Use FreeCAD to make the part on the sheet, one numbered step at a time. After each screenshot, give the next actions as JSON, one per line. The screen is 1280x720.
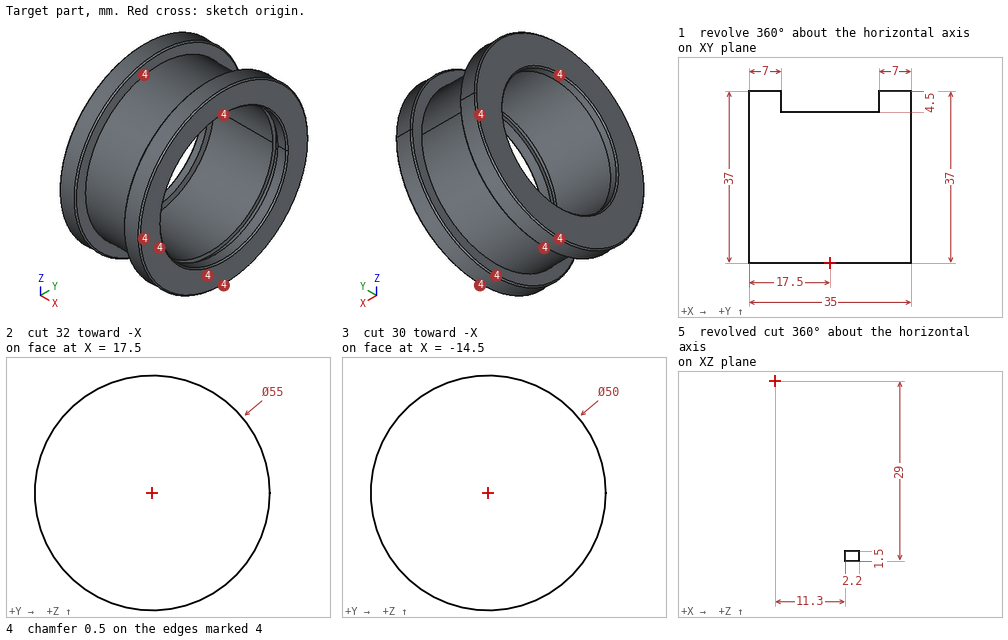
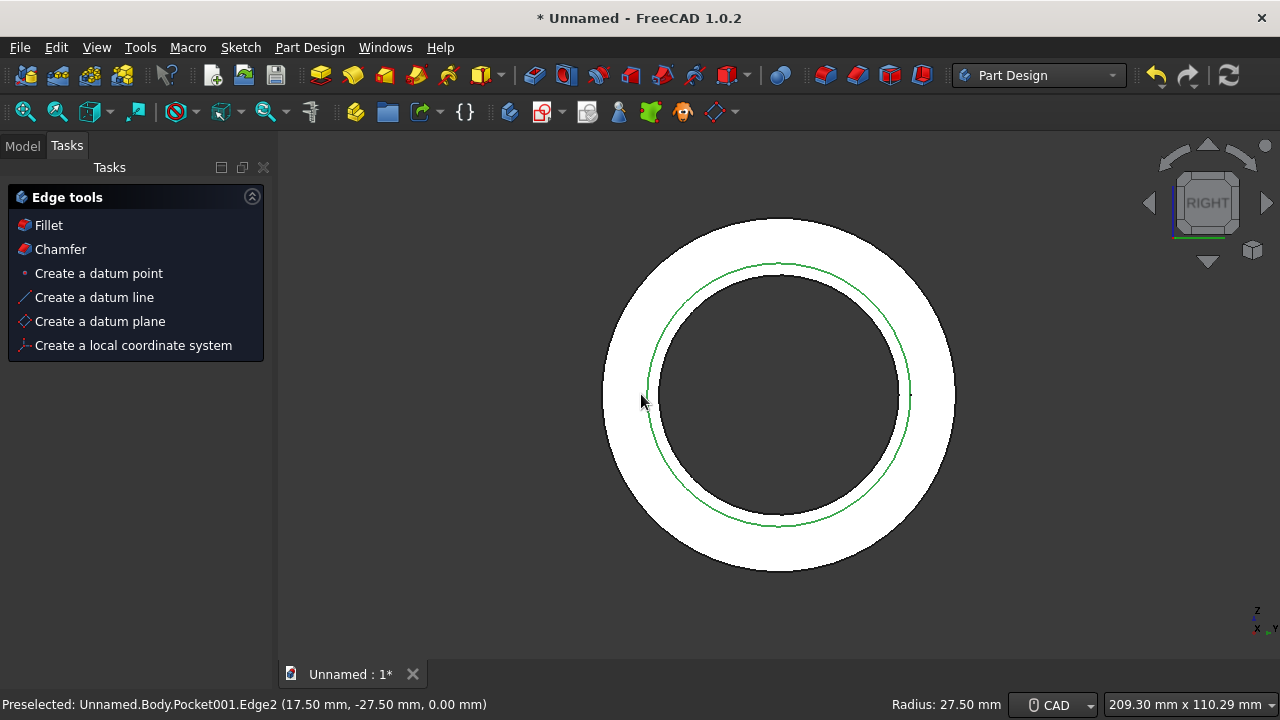
{"action": "left_click", "coordinate": [724, 562], "text": "ctrl"}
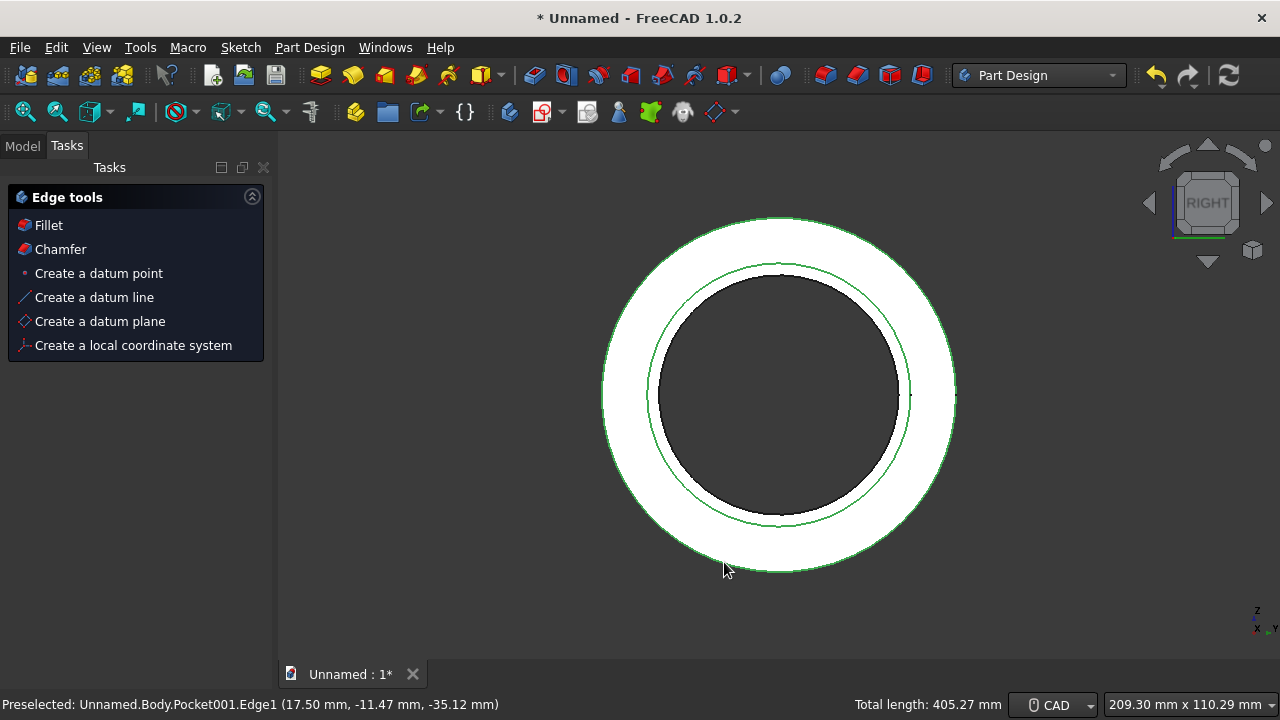
{"action": "key", "text": "0"}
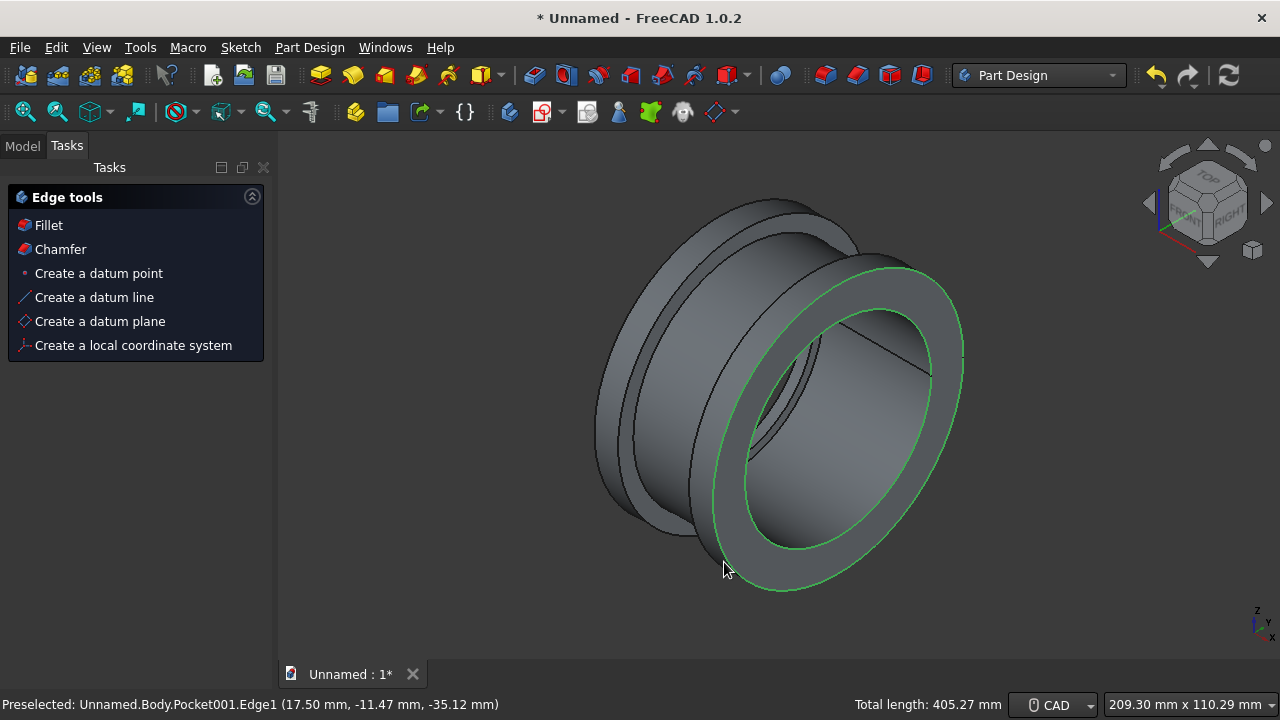
{"action": "left_click", "coordinate": [618, 446], "text": "ctrl"}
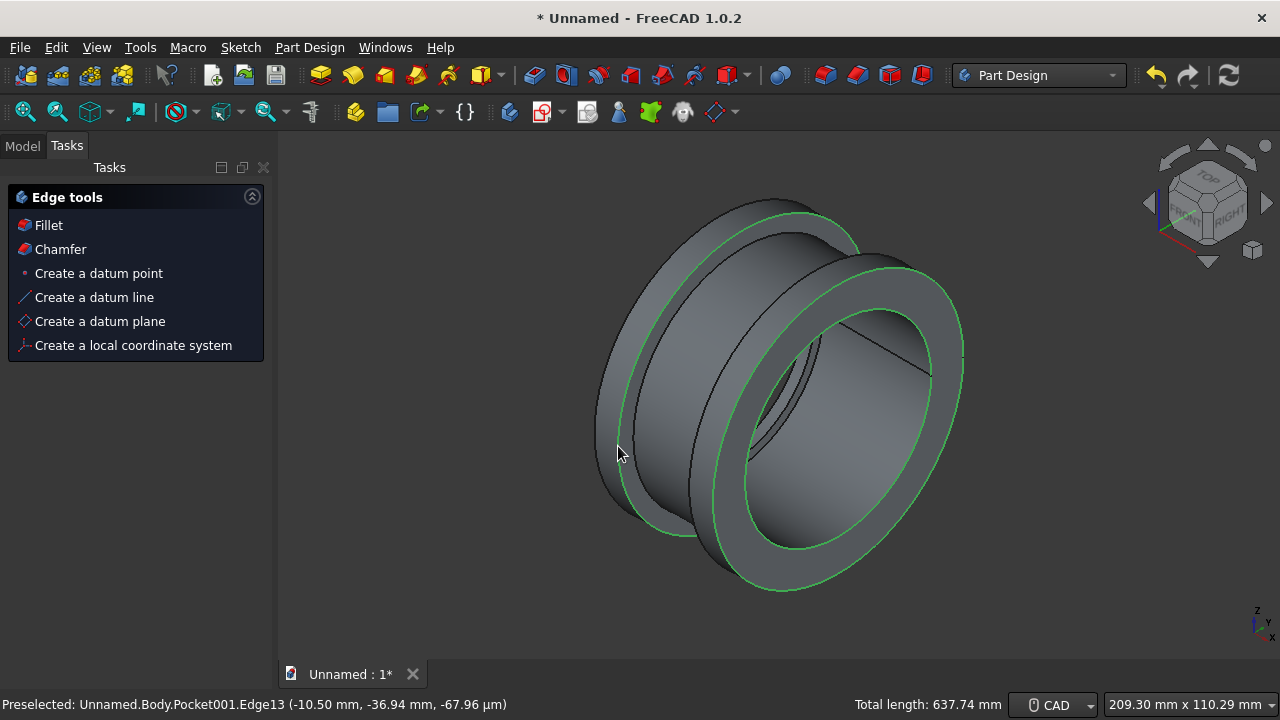
{"action": "key", "text": "2"}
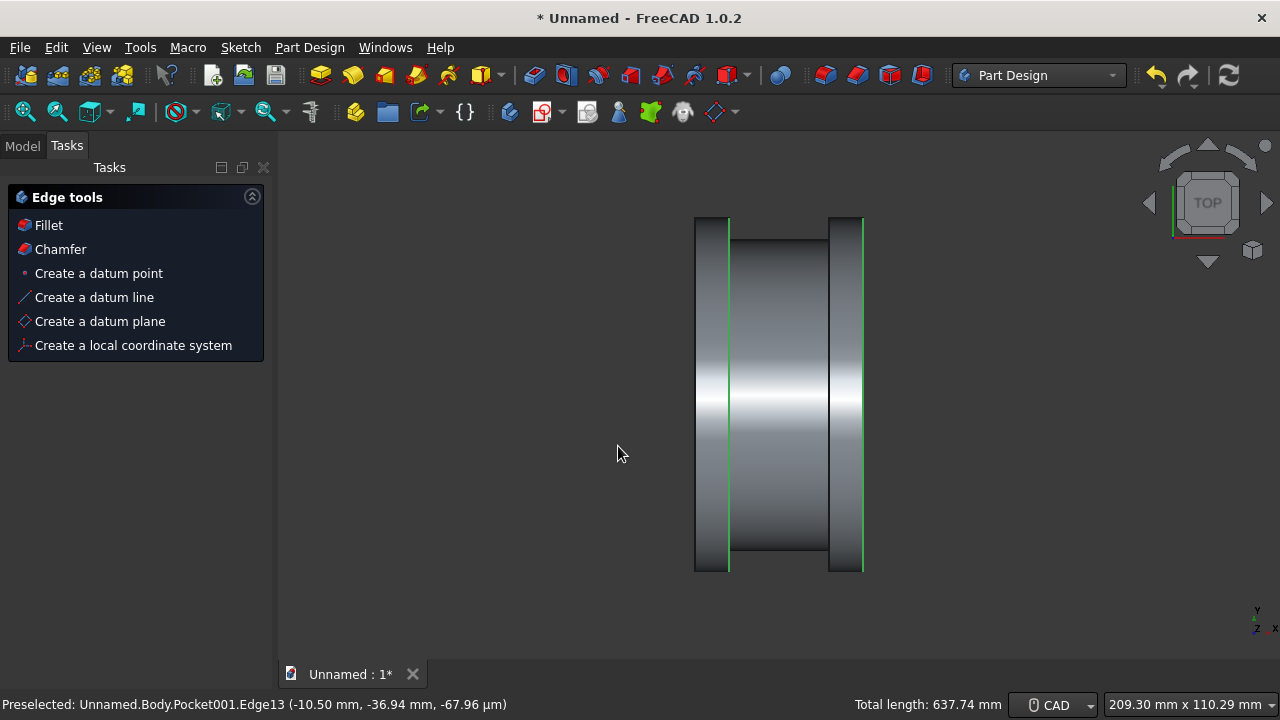
{"action": "left_click", "coordinate": [695, 537], "text": "ctrl"}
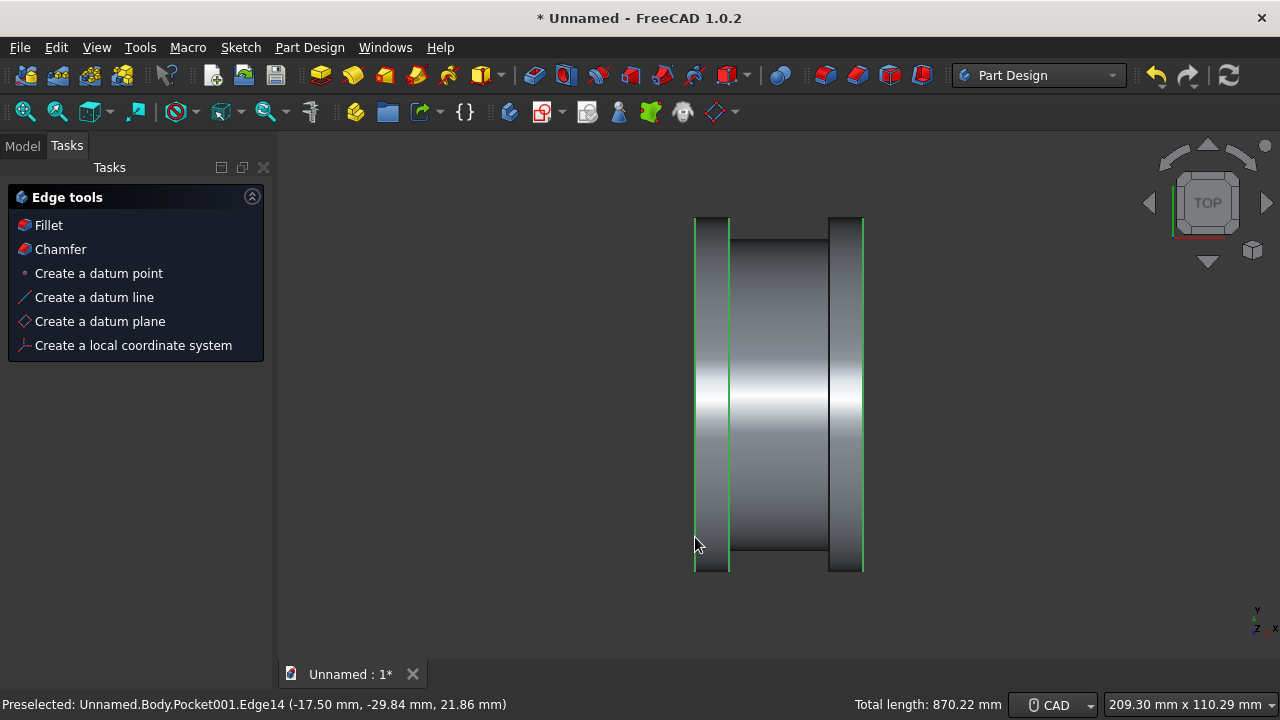
{"action": "left_click", "coordinate": [829, 537], "text": "ctrl"}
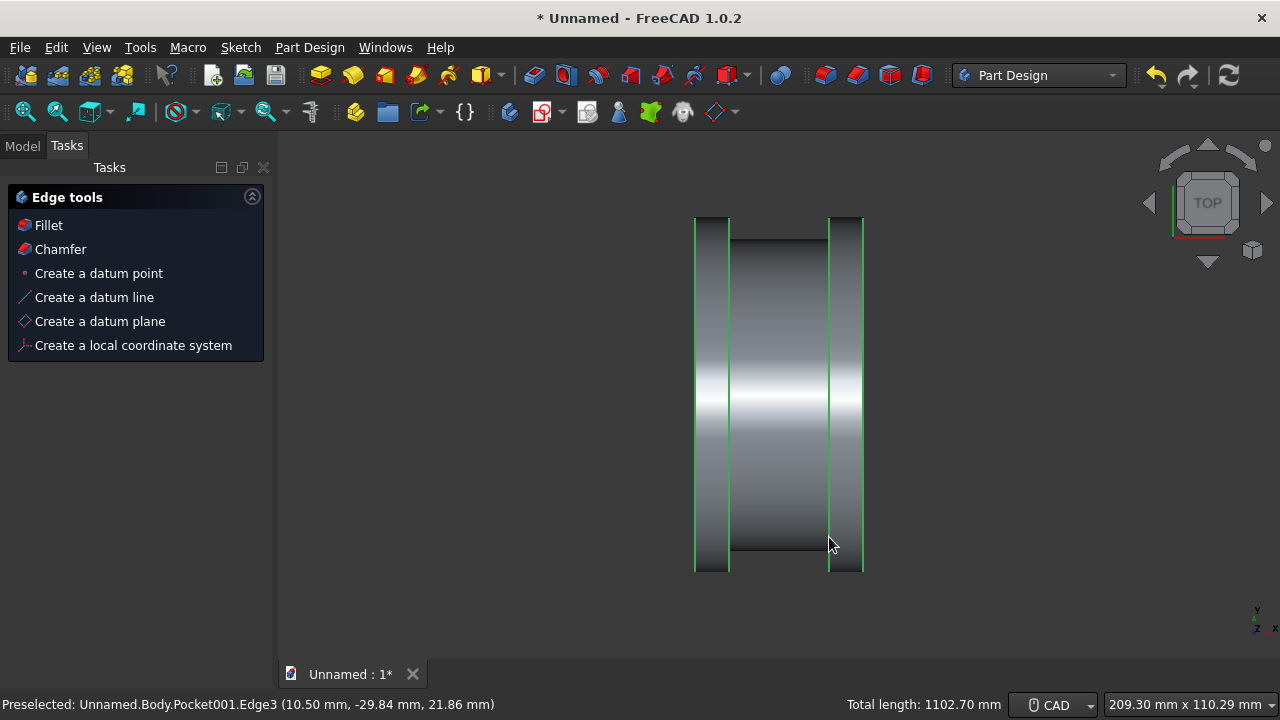
{"action": "key", "text": "1"}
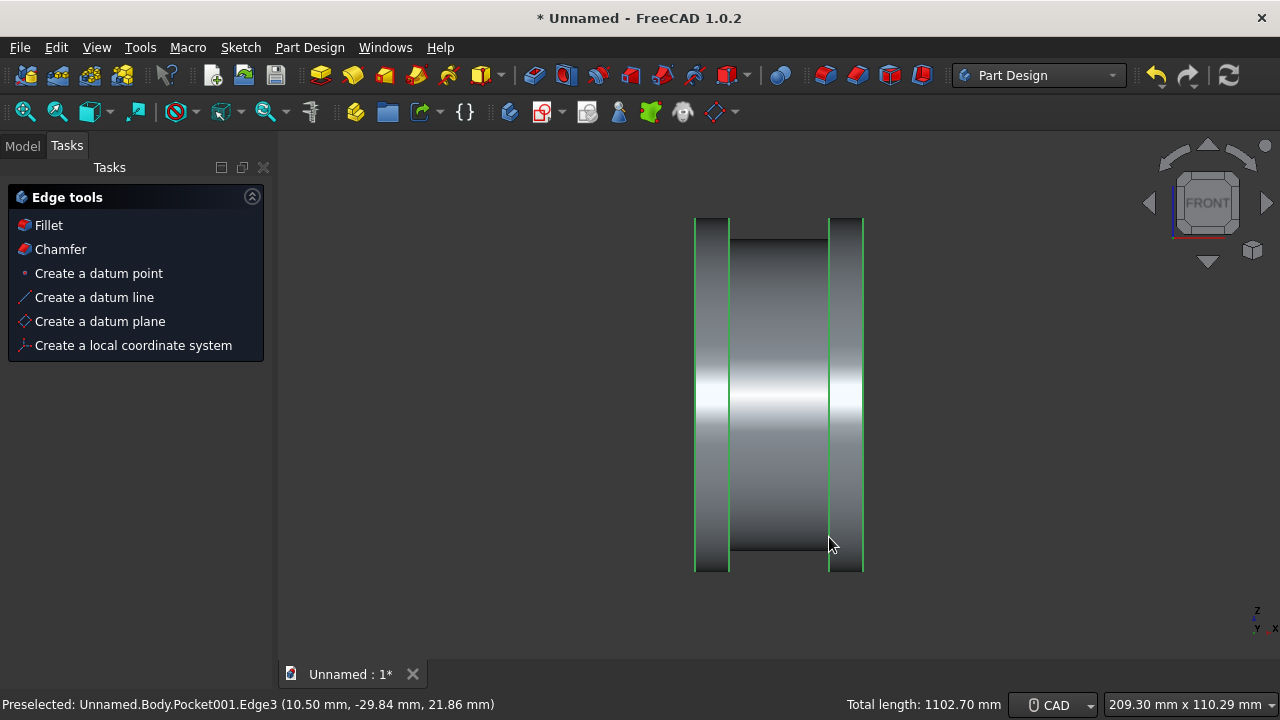
{"action": "key", "text": "3"}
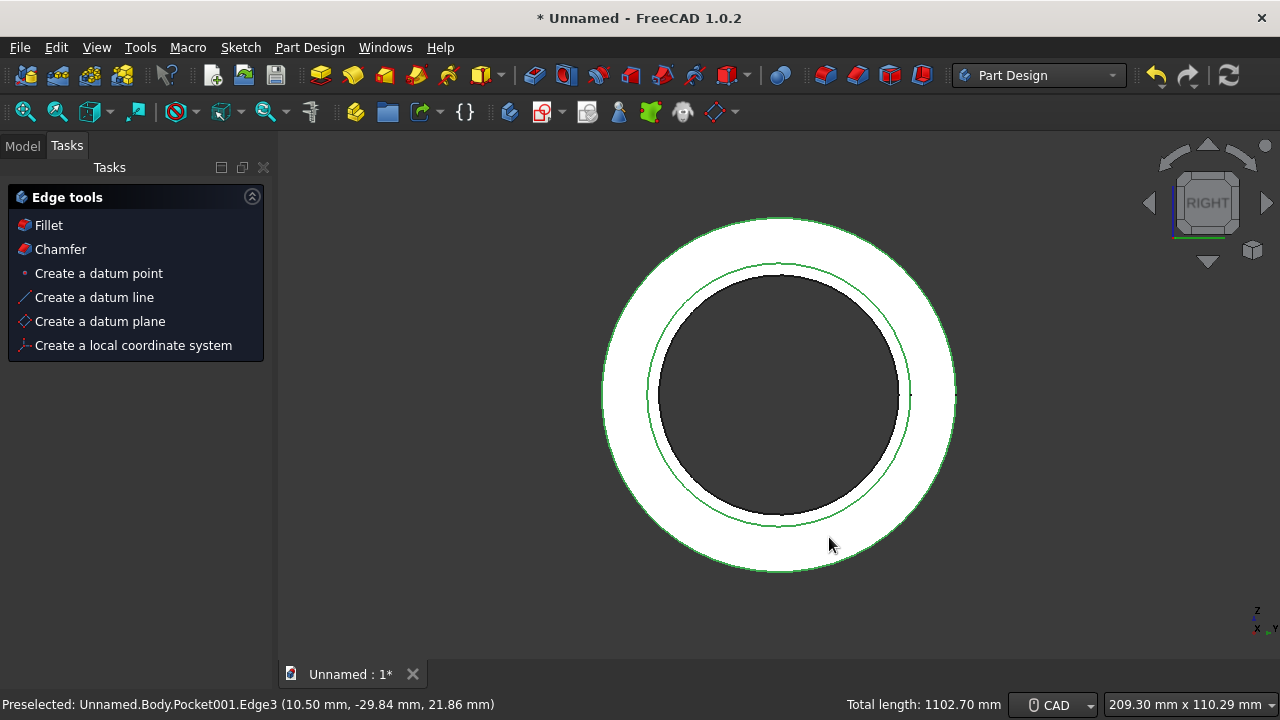
{"action": "key", "text": "5"}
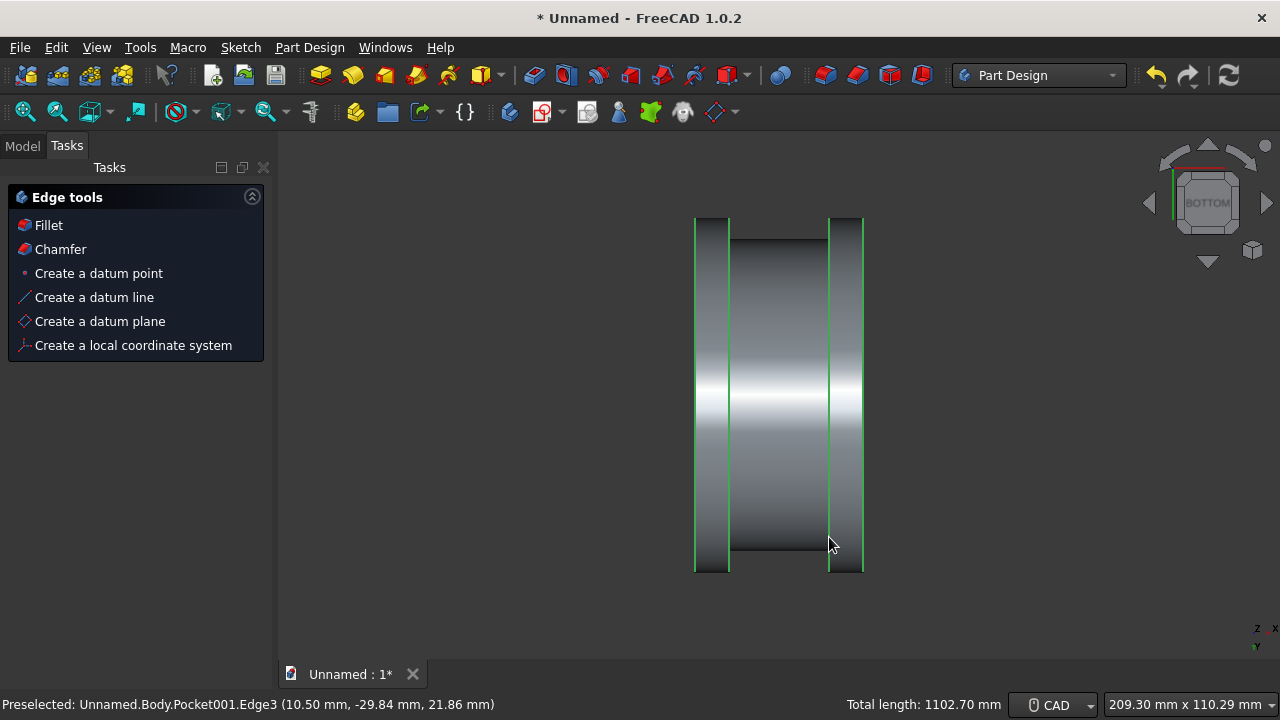
{"action": "key", "text": "4"}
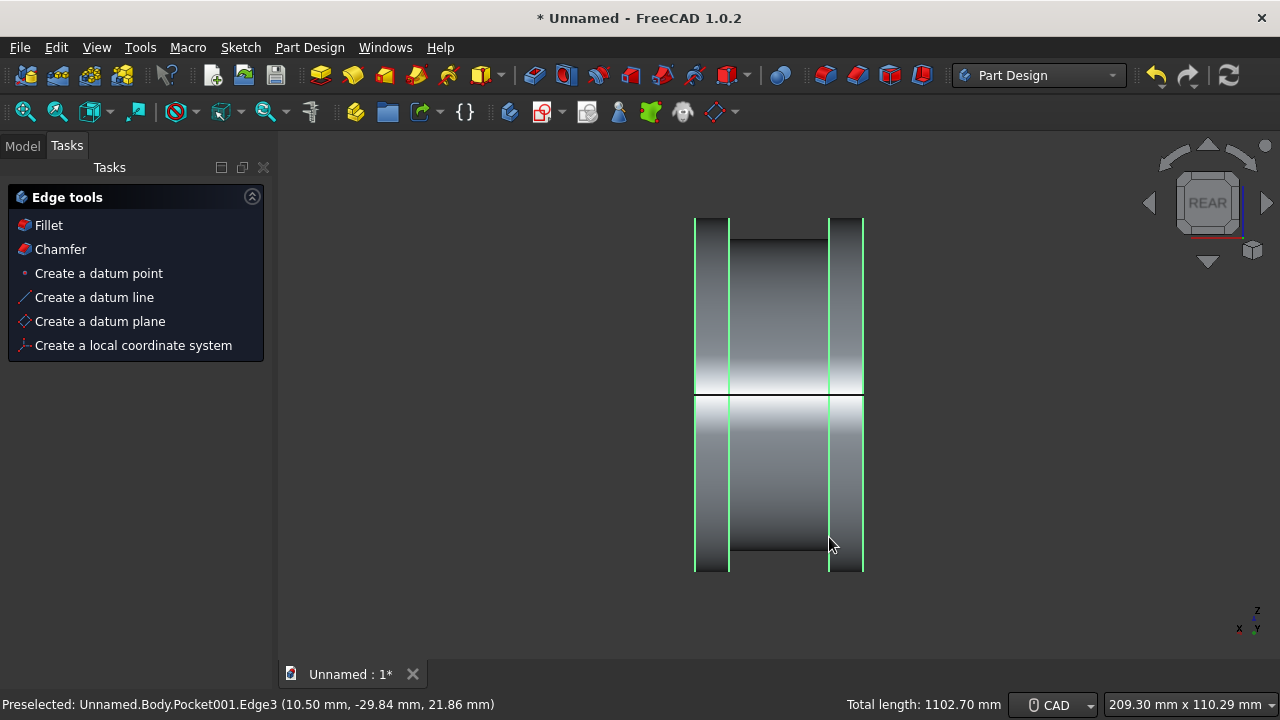
{"action": "key", "text": "6"}